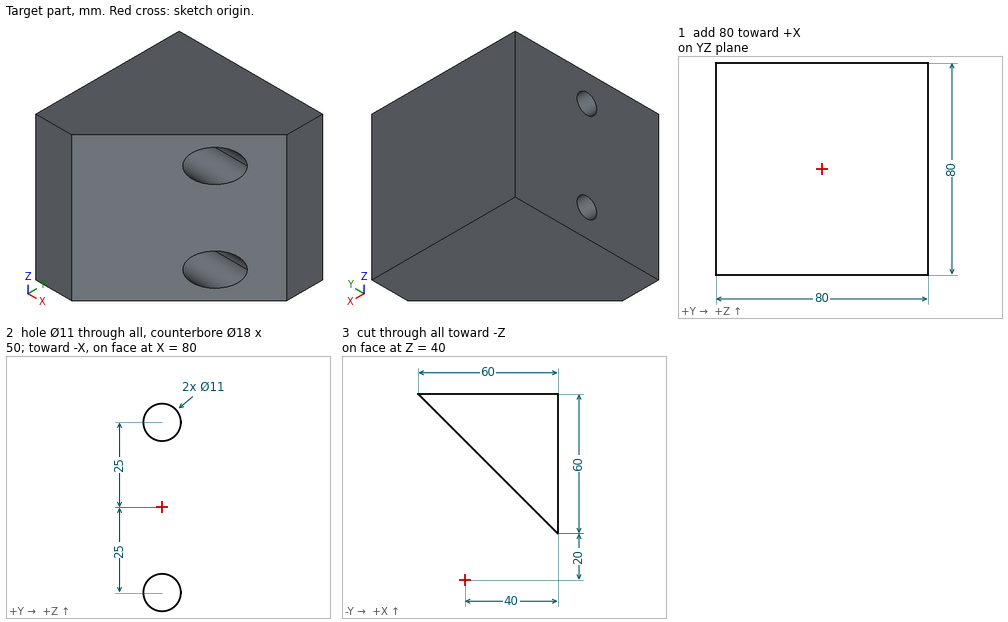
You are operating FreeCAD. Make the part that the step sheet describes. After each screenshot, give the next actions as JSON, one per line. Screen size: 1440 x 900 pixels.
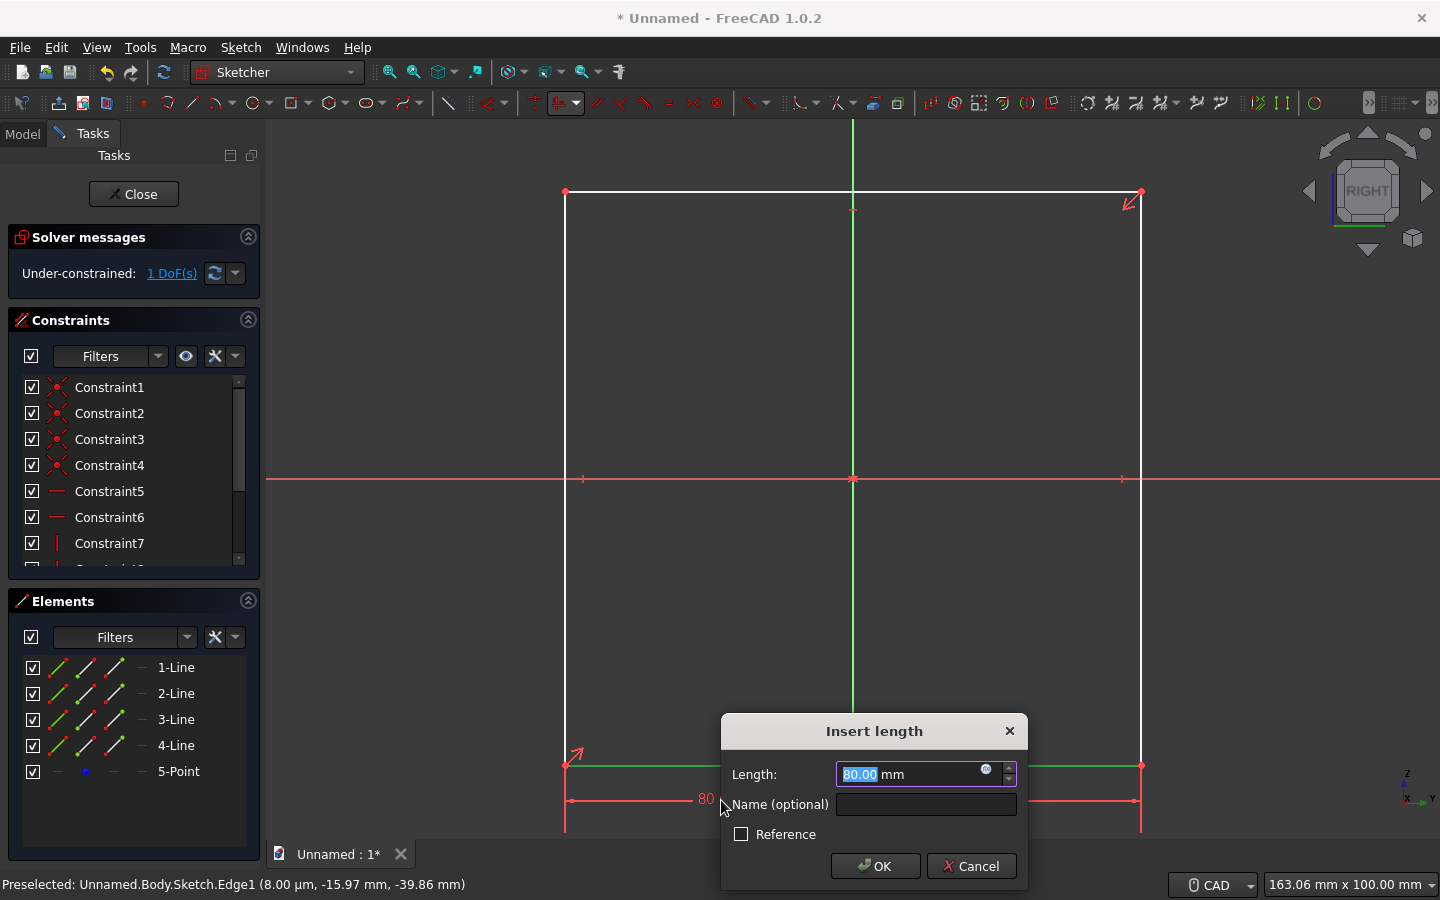
{"action": "type", "text": "80"}
{"action": "key", "text": "Return"}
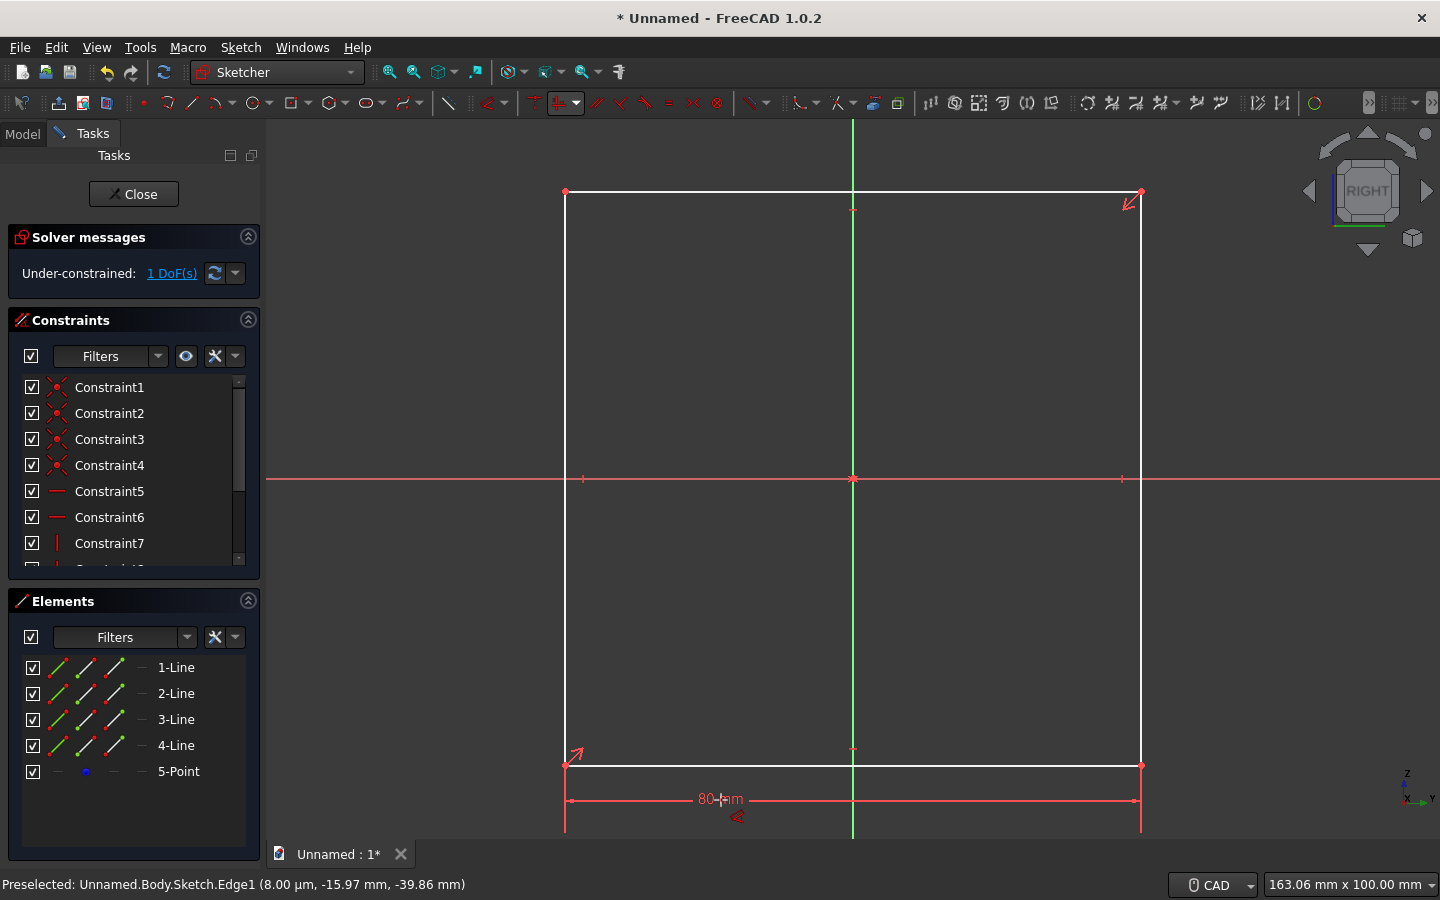
{"action": "left_click", "coordinate": [1141, 594]}
{"action": "left_click", "coordinate": [1175, 347]}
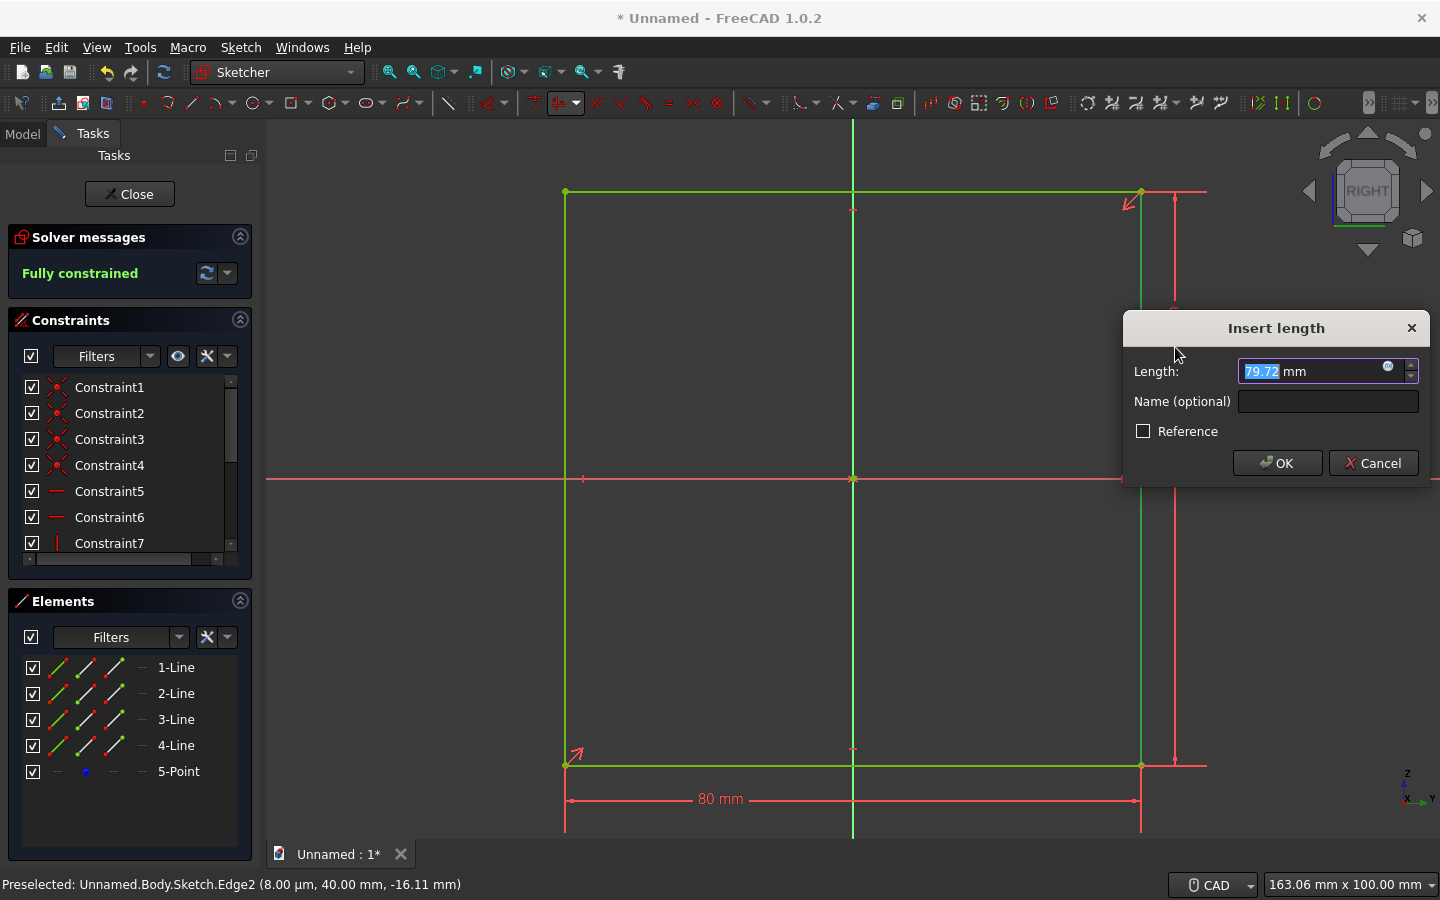
{"action": "type", "text": "80"}
{"action": "key", "text": "Return"}
{"action": "key", "text": "Escape"}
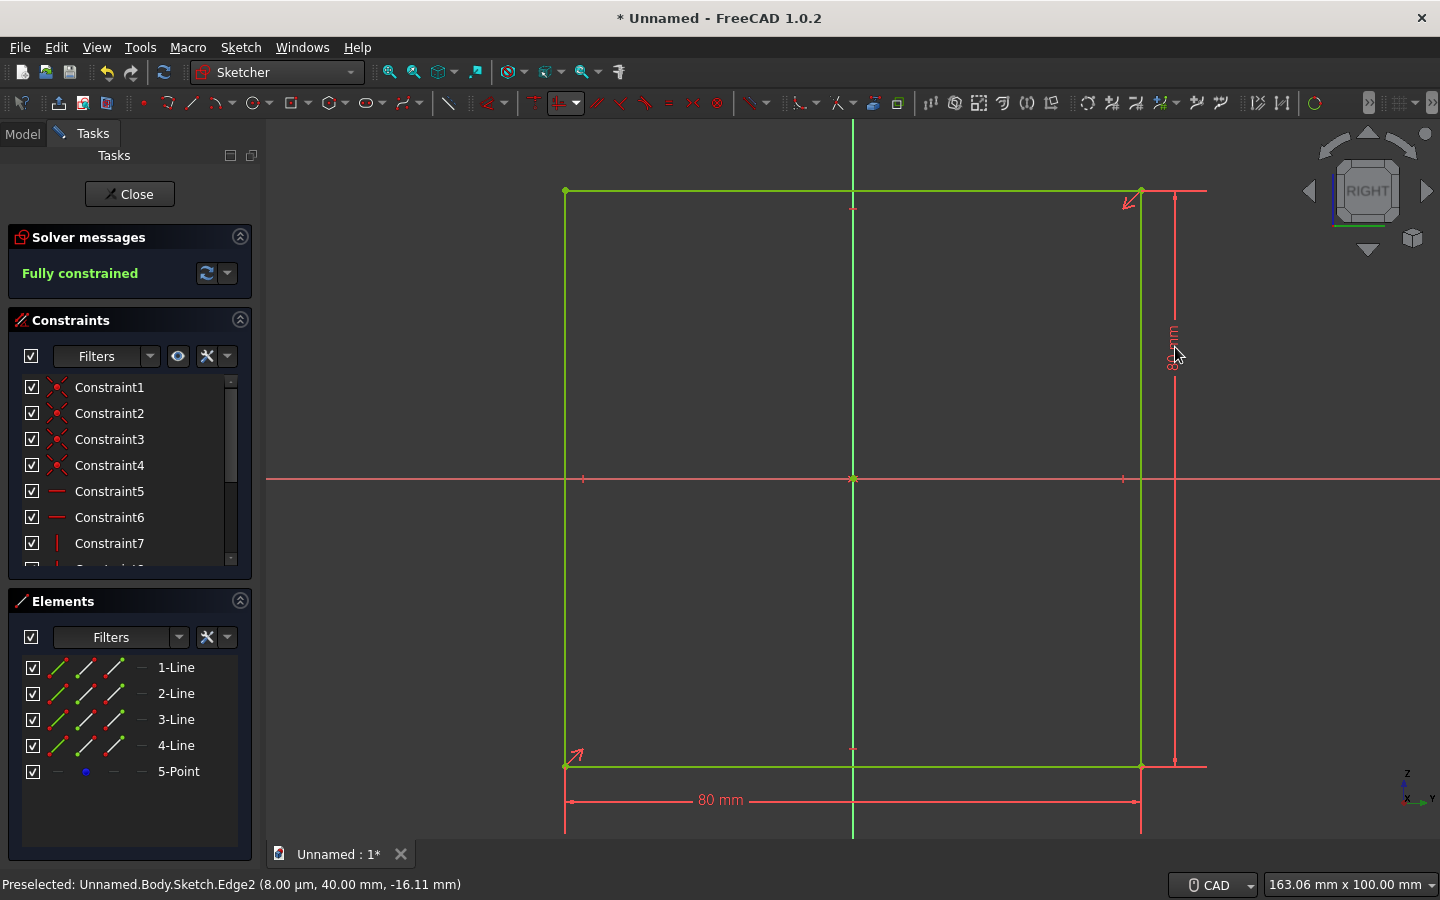
{"action": "left_click", "coordinate": [130, 194]}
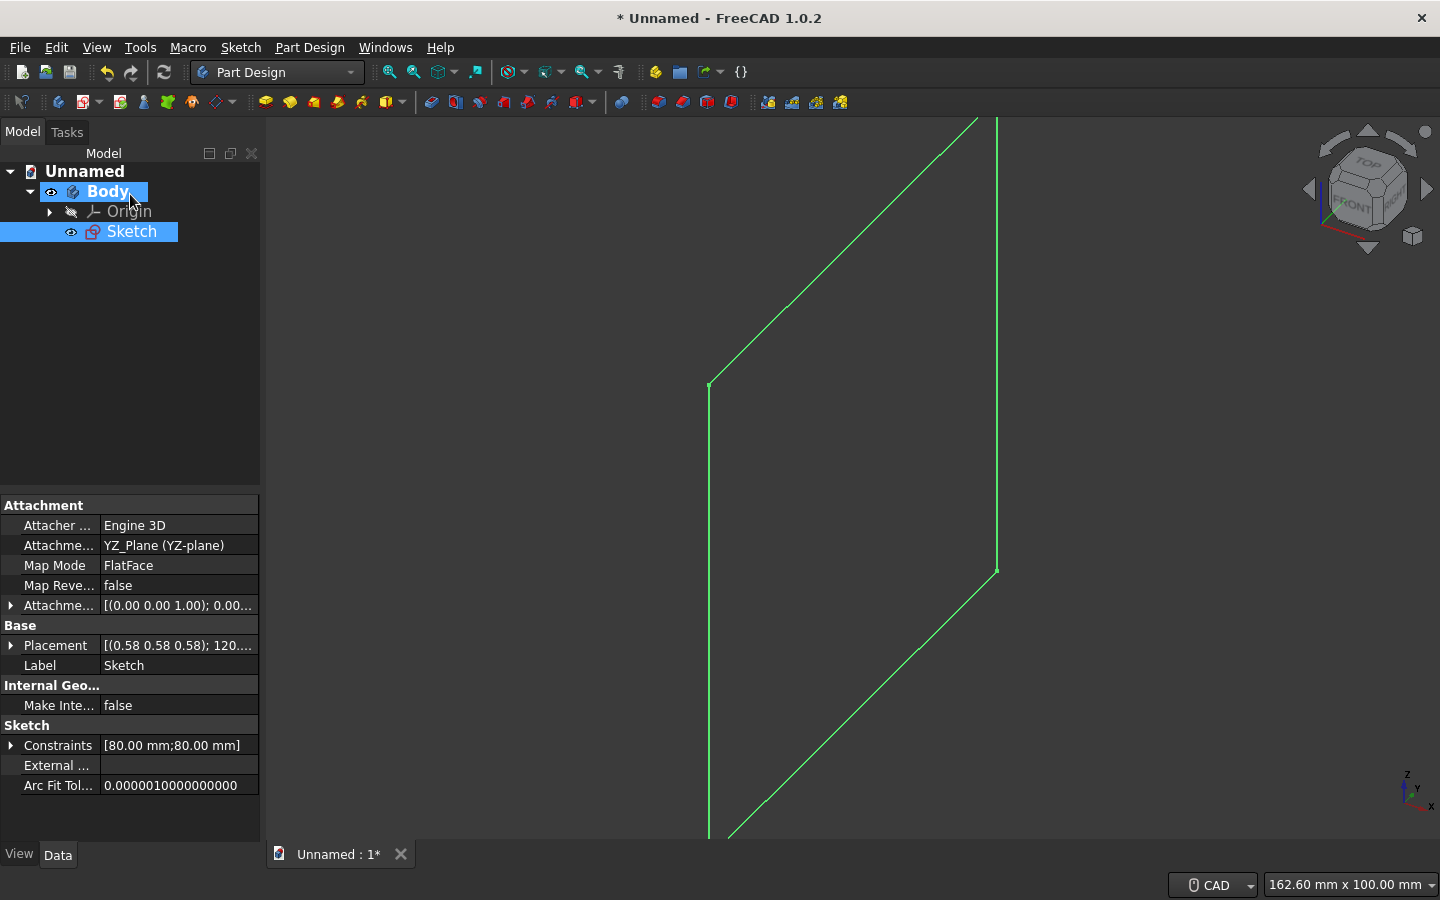
{"action": "left_click", "coordinate": [266, 102]}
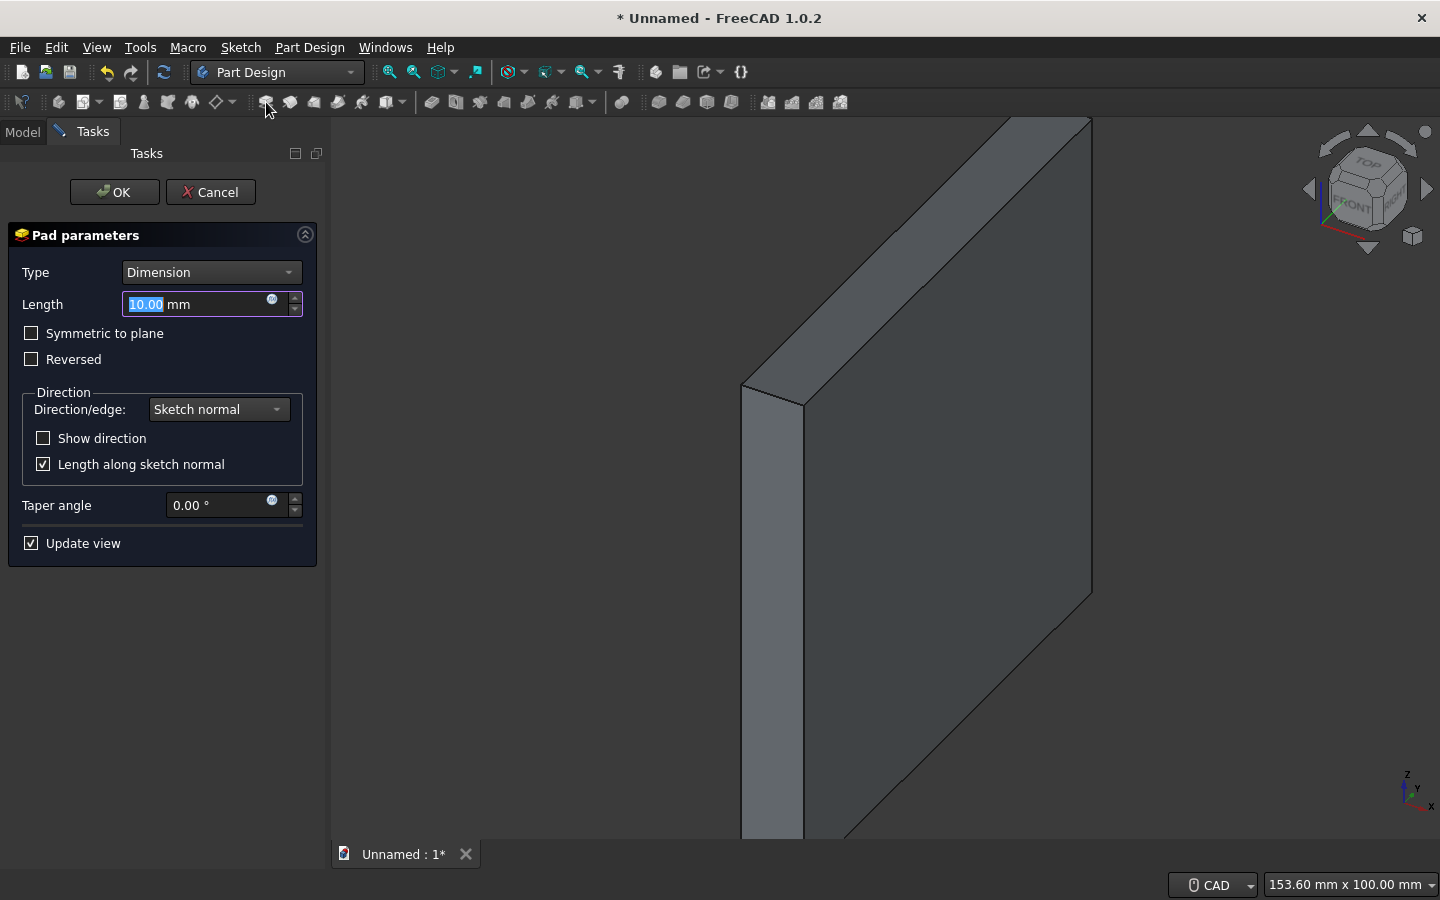
{"action": "type", "text": "80"}
{"action": "key", "text": "Tab"}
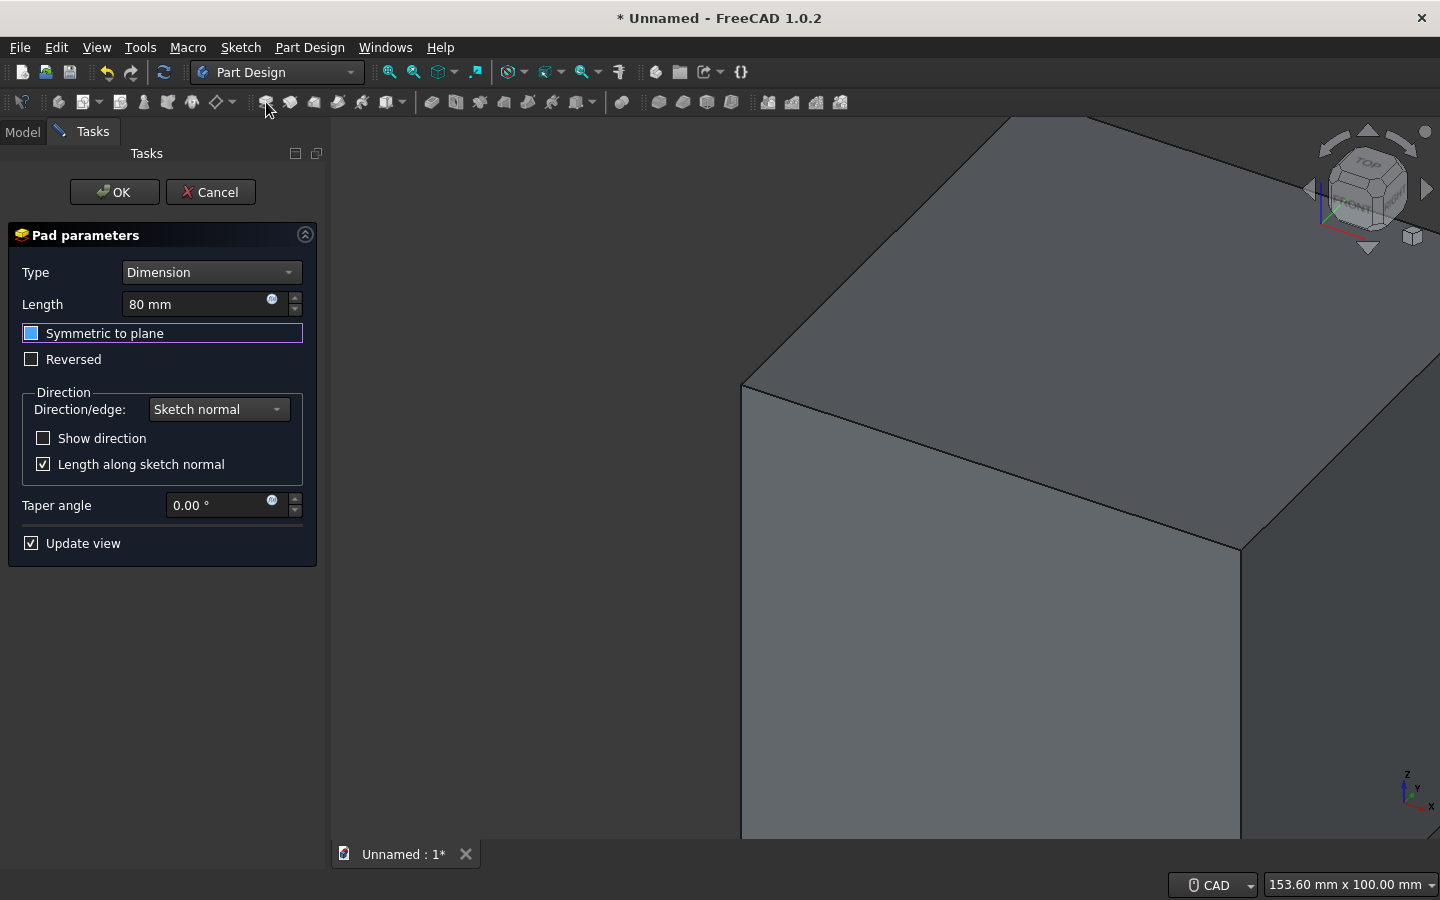
{"action": "left_click", "coordinate": [115, 192]}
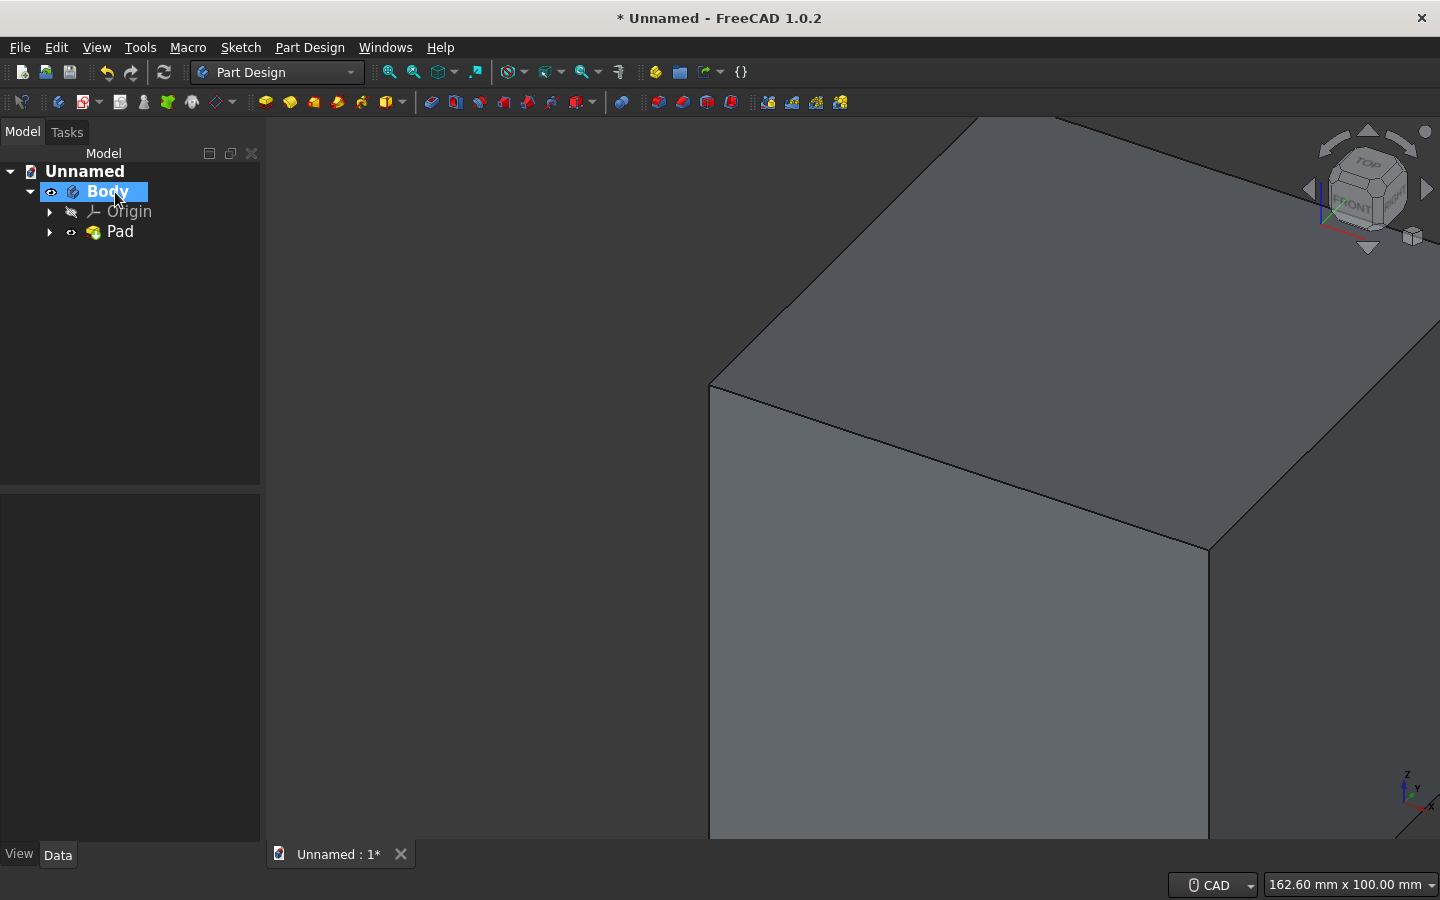
{"action": "left_click", "coordinate": [390, 72]}